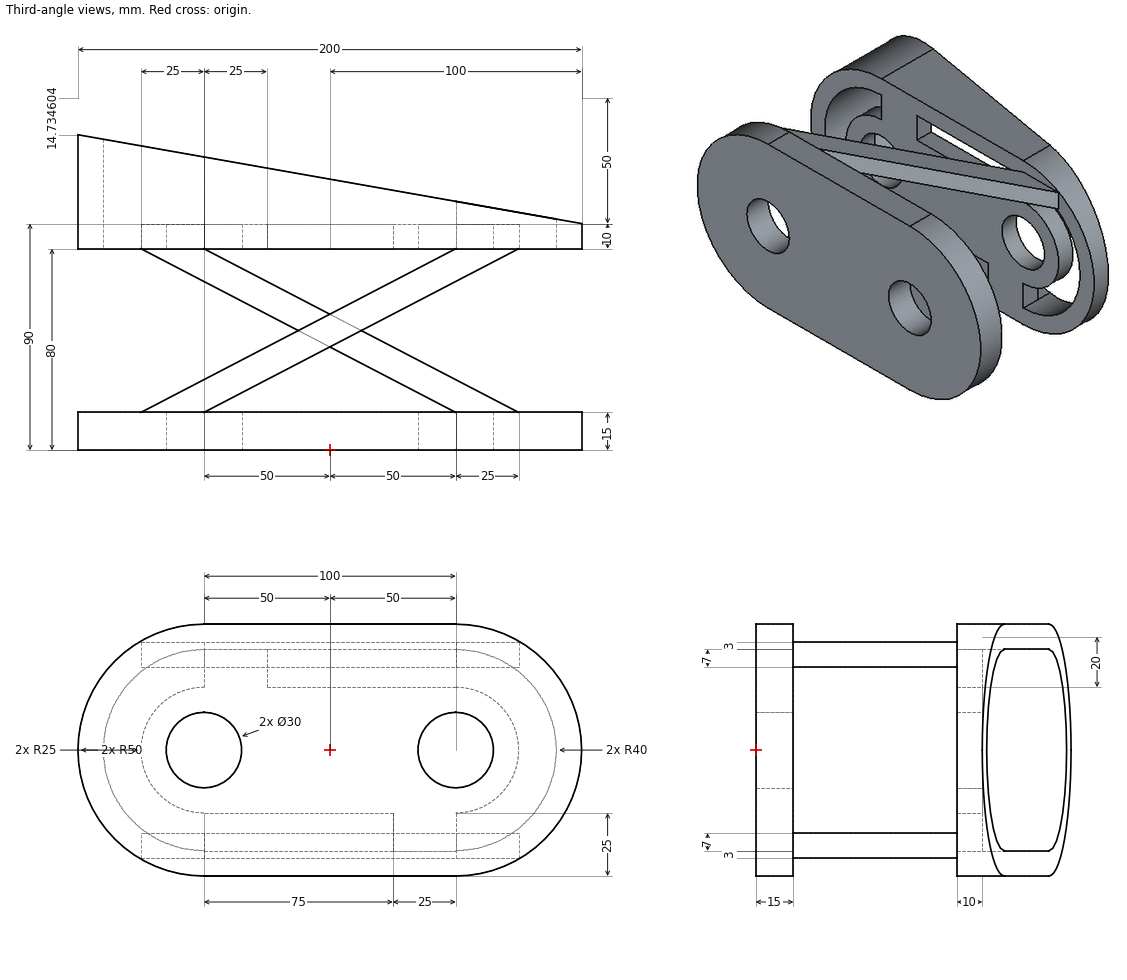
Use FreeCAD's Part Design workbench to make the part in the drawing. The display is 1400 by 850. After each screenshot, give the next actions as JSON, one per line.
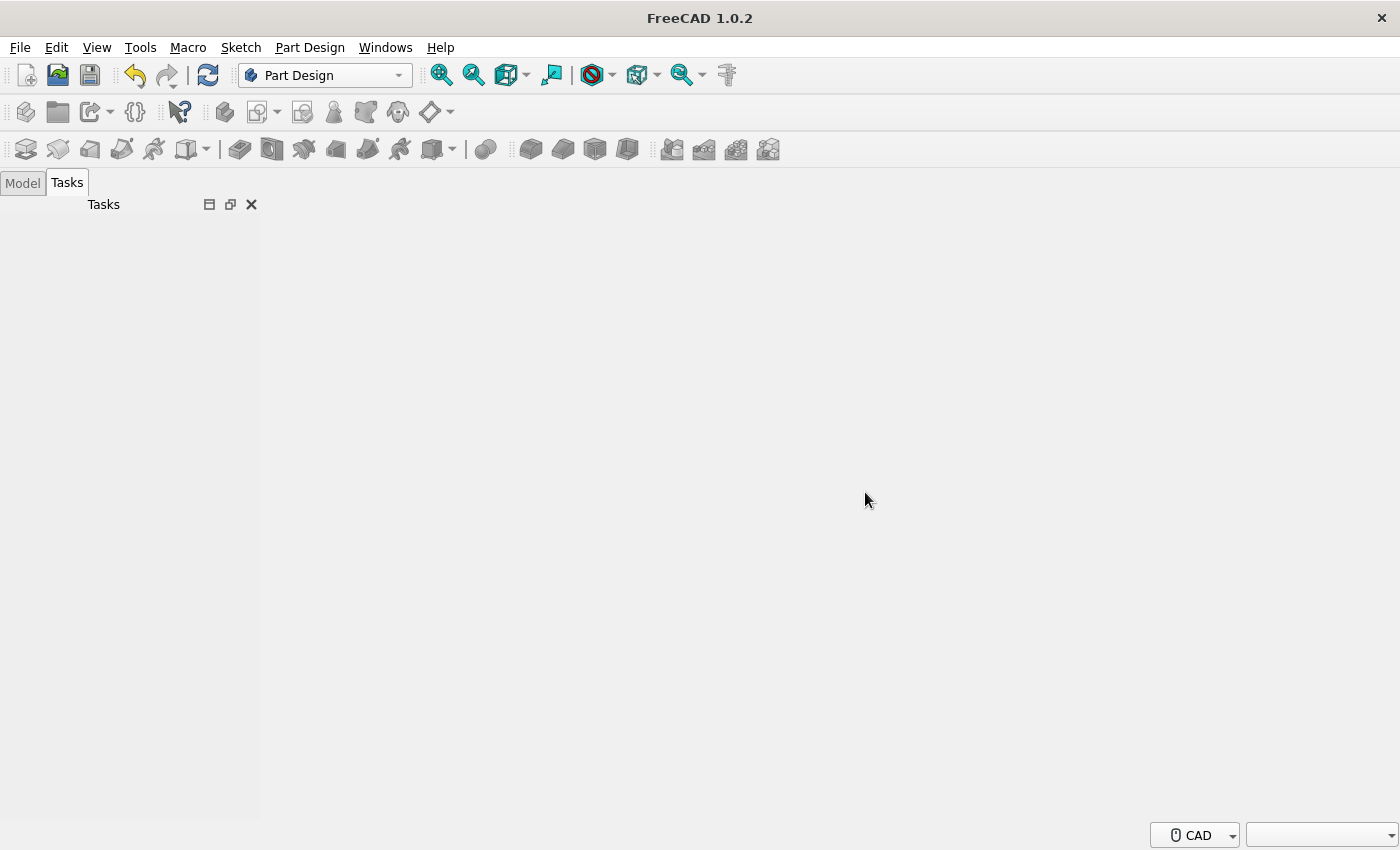
{"action": "left_click", "coordinate": [26, 76]}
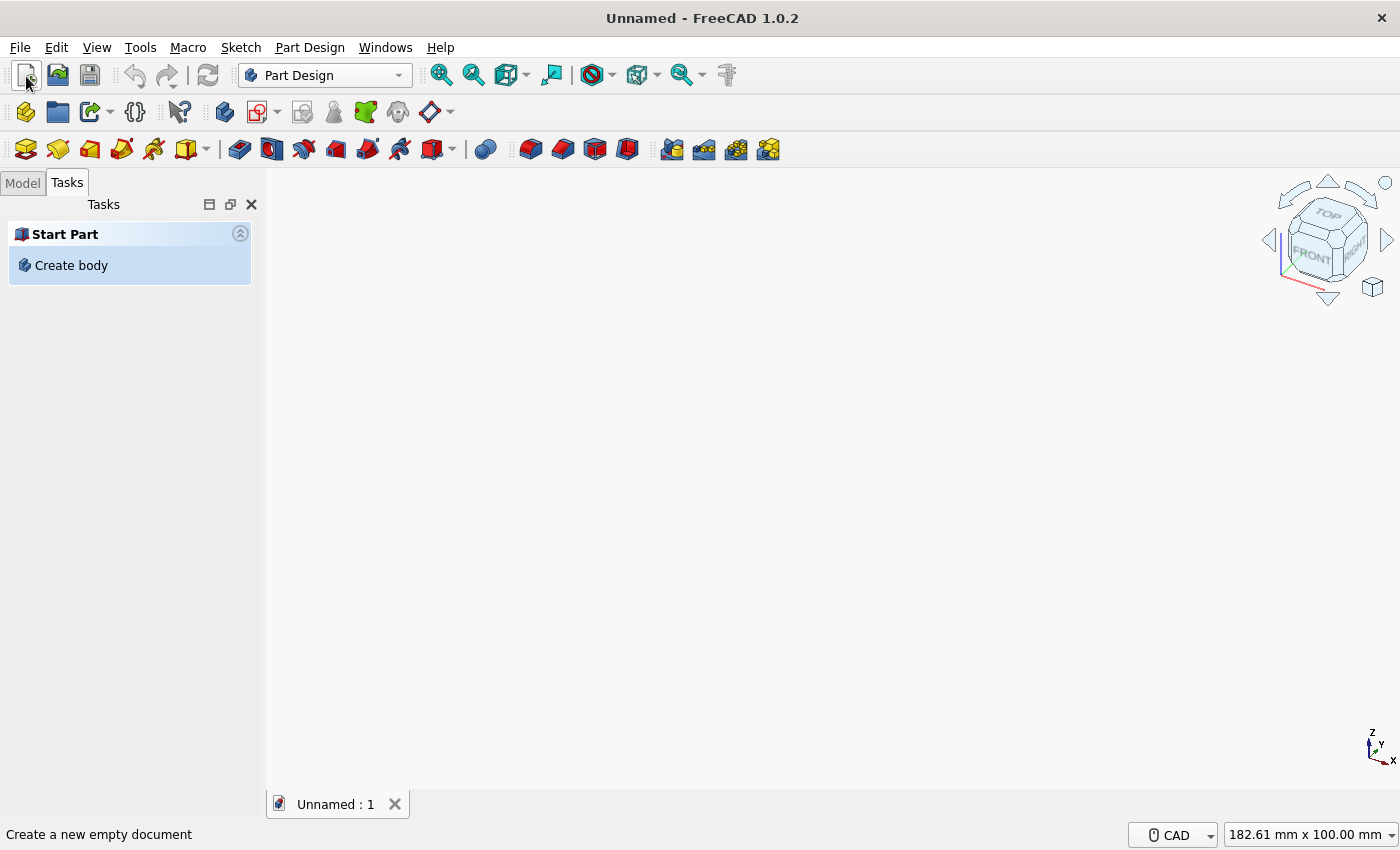
{"action": "left_click", "coordinate": [258, 112]}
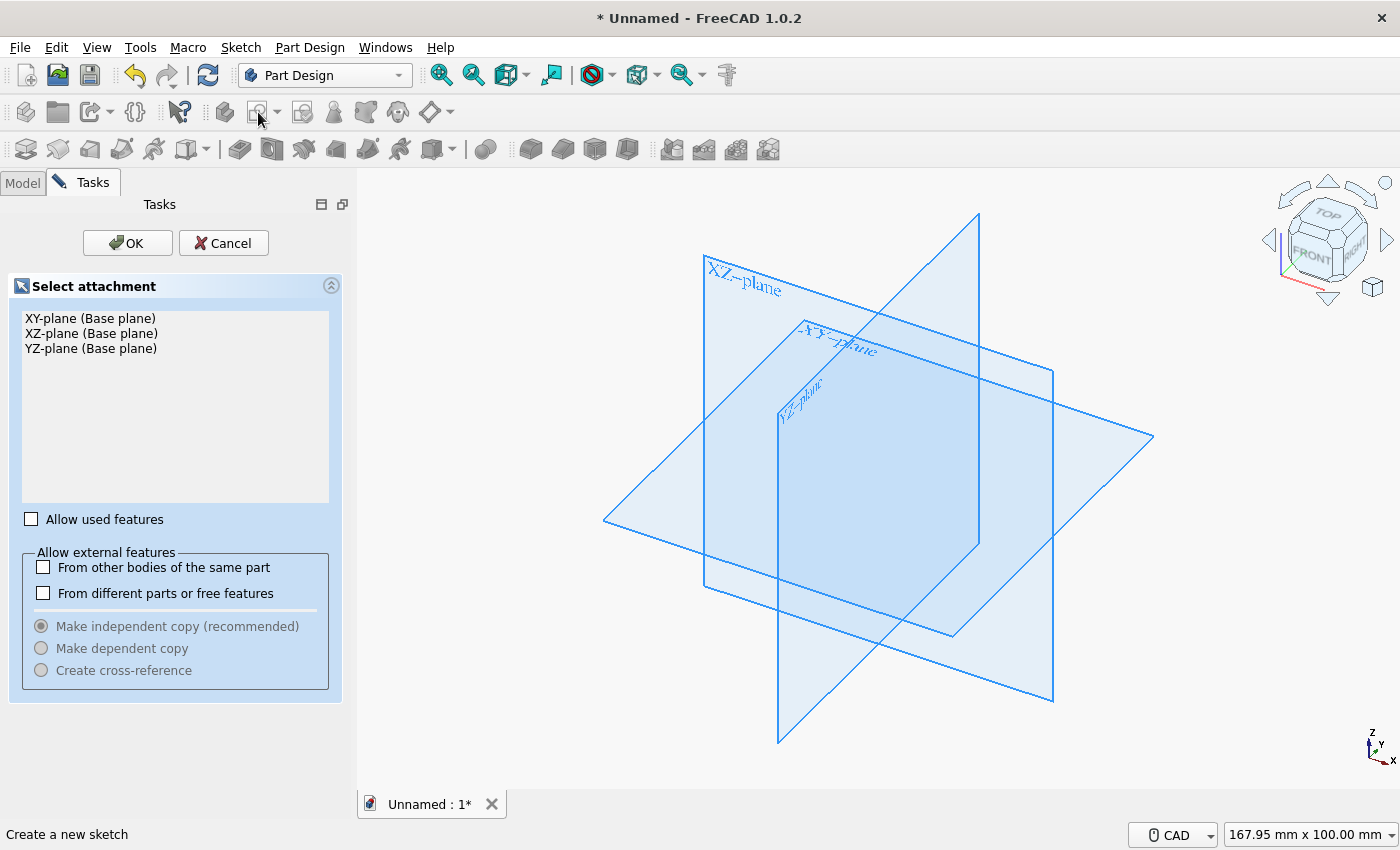
{"action": "left_click", "coordinate": [82, 334]}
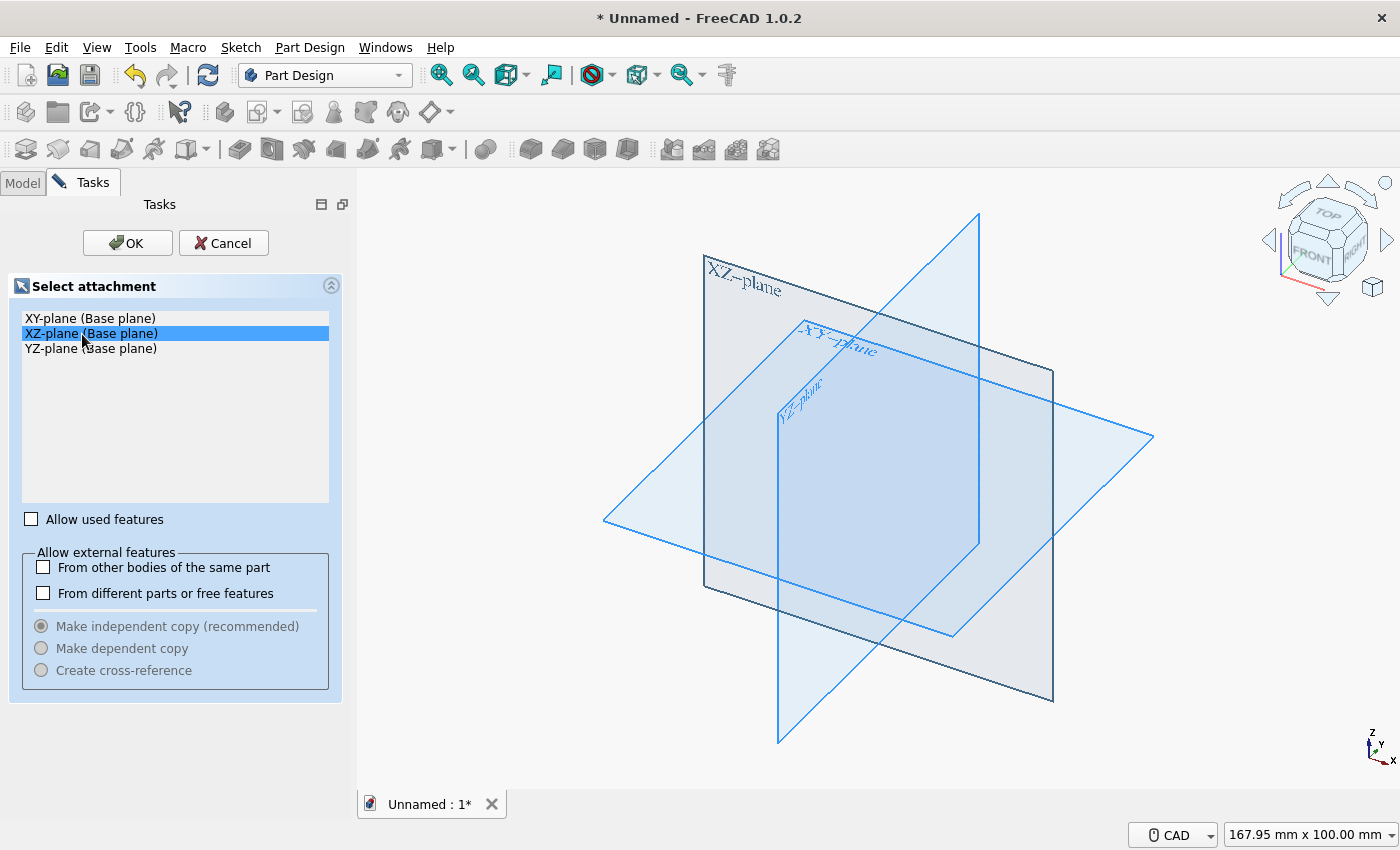
{"action": "left_click", "coordinate": [128, 243]}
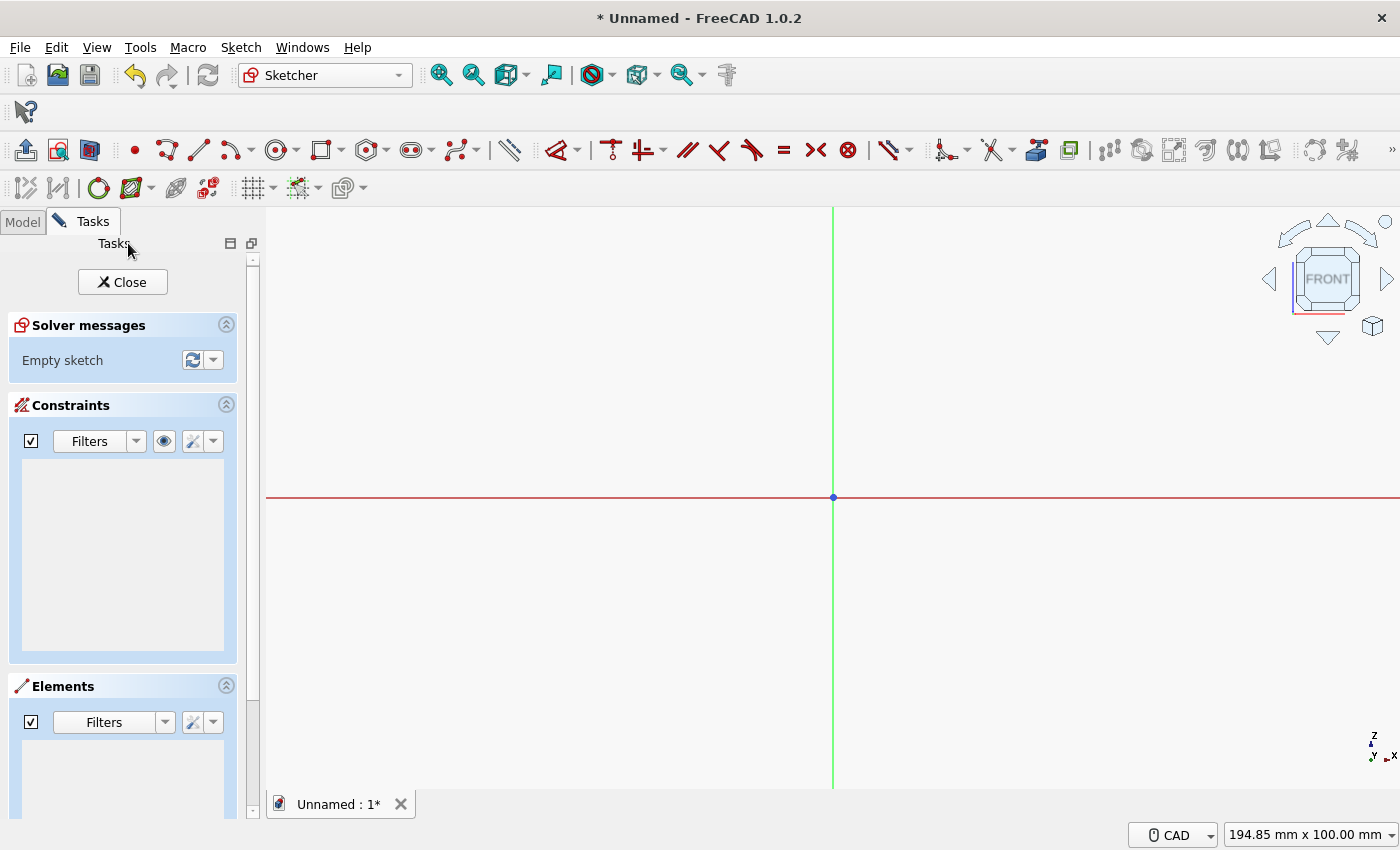
{"action": "scroll", "coordinate": [681, 498], "scroll_direction": "down", "scroll_amount": 3}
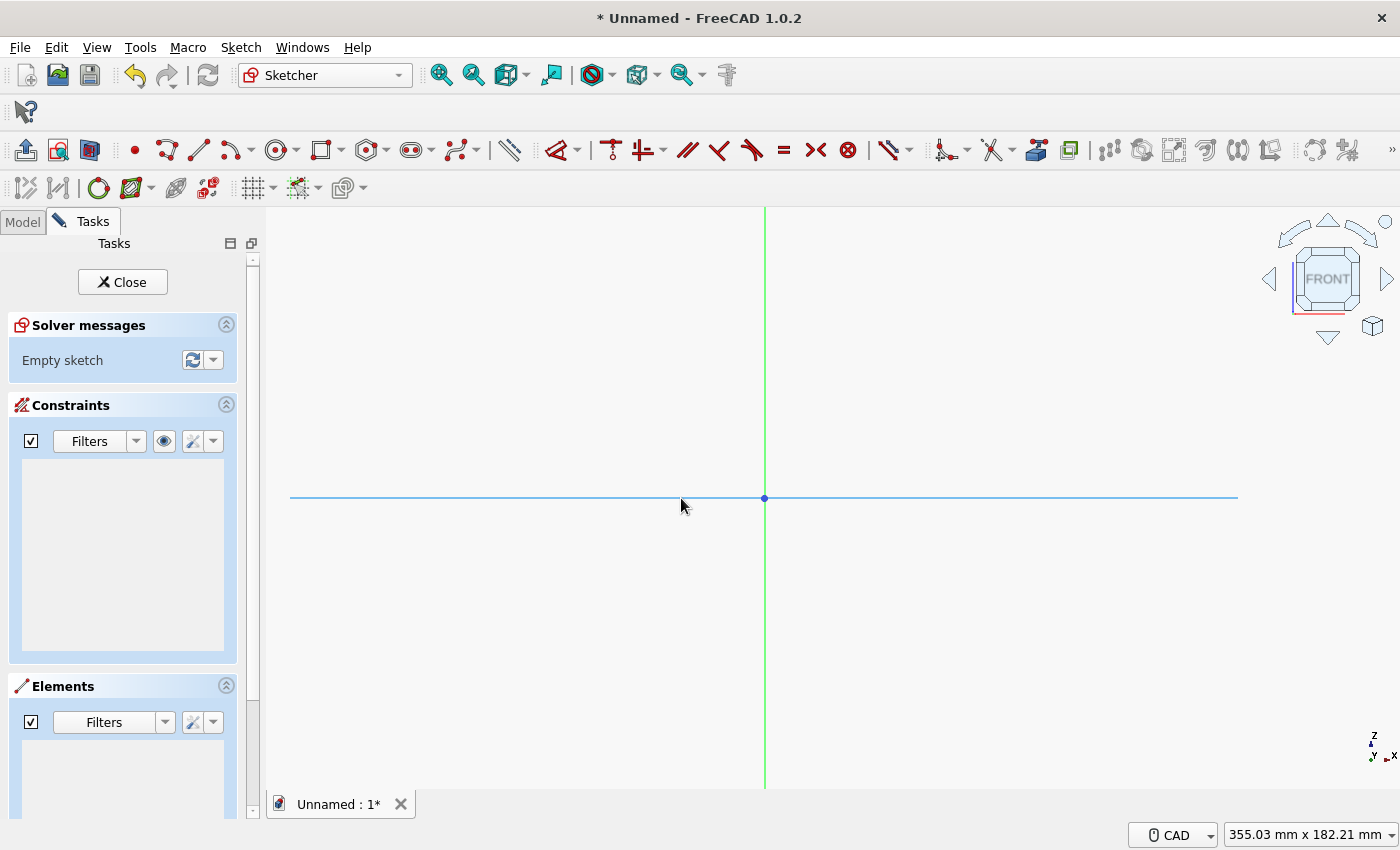
{"action": "left_click", "coordinate": [412, 150]}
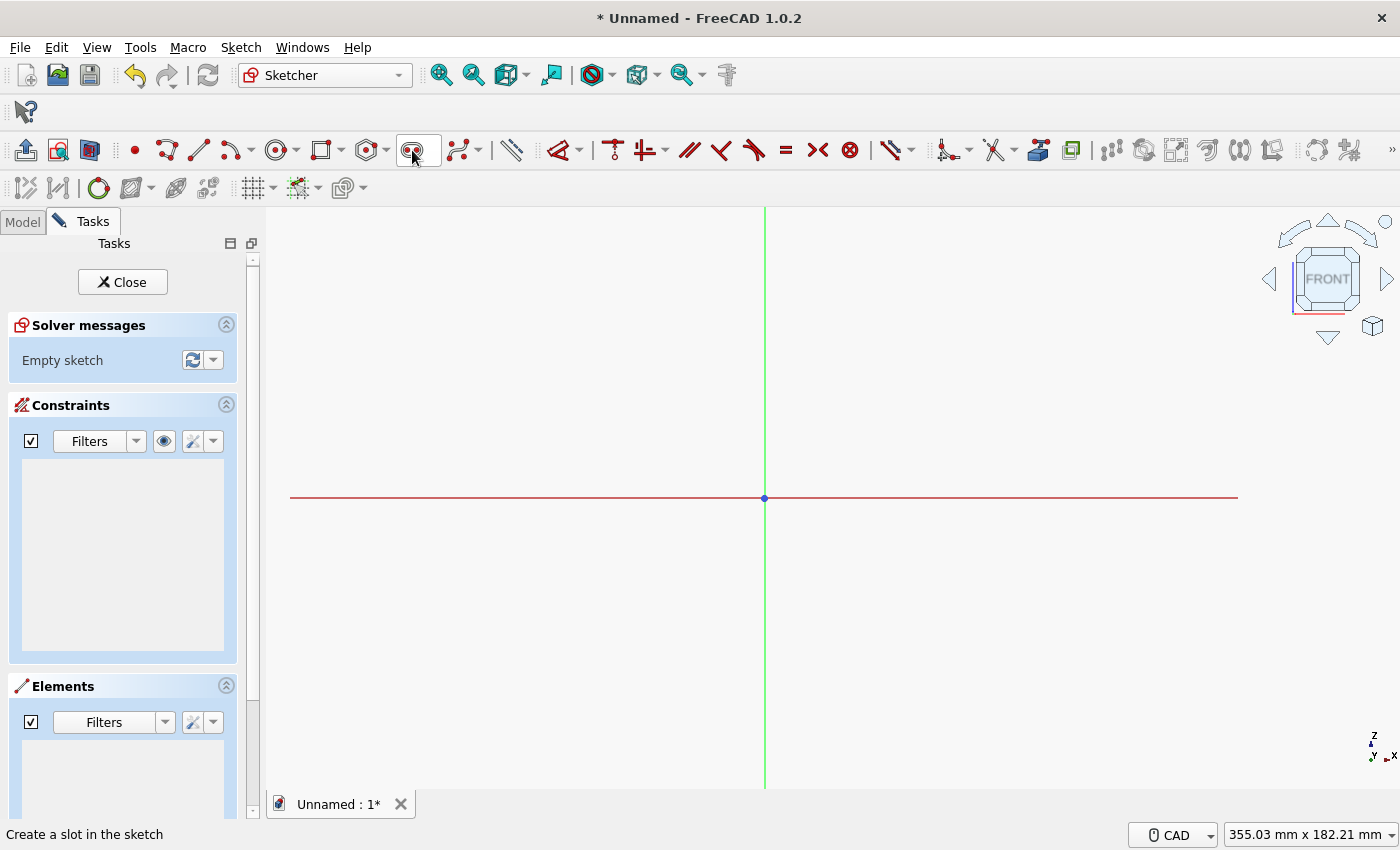
{"action": "left_click", "coordinate": [605, 498]}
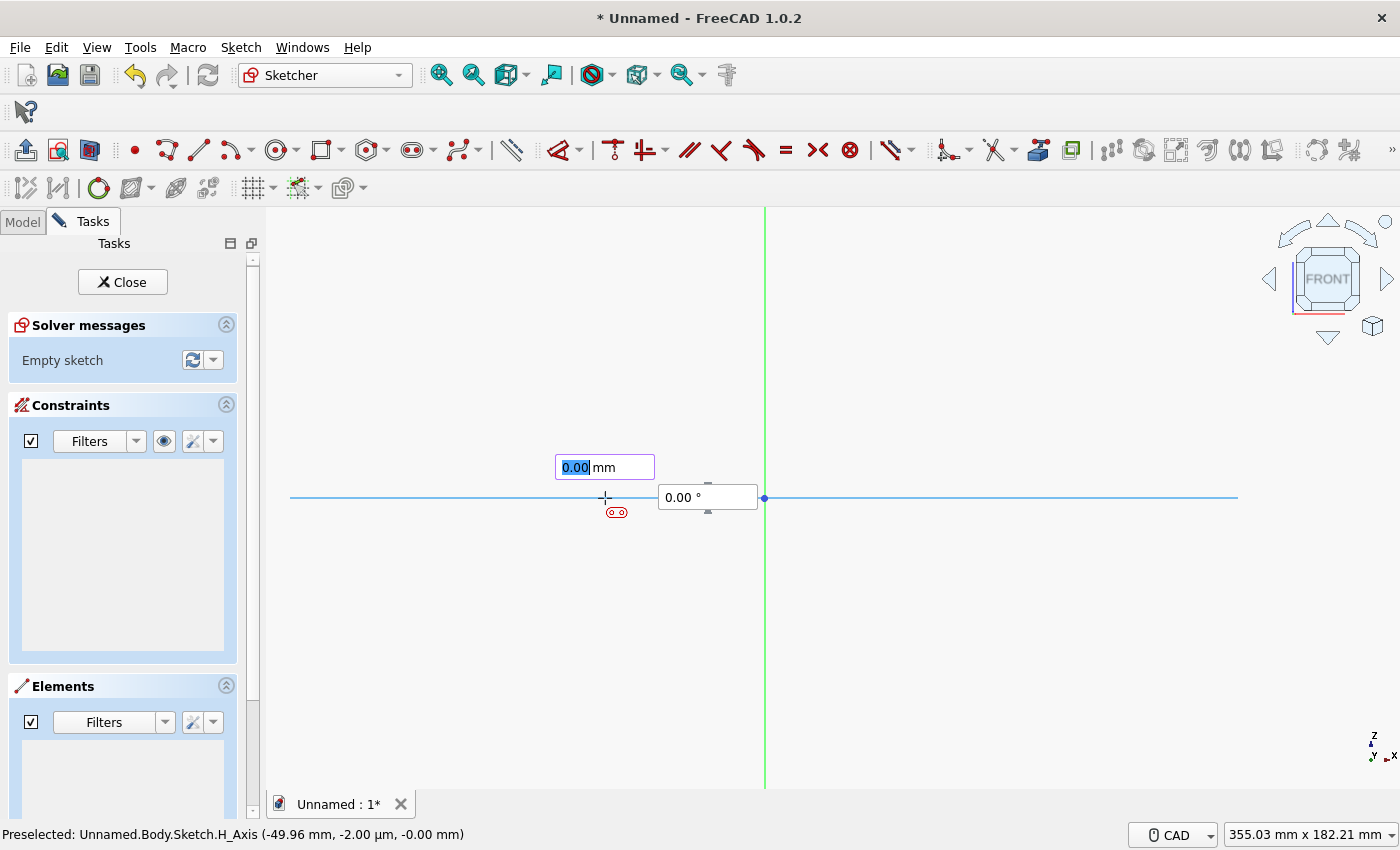
{"action": "left_click", "coordinate": [924, 489]}